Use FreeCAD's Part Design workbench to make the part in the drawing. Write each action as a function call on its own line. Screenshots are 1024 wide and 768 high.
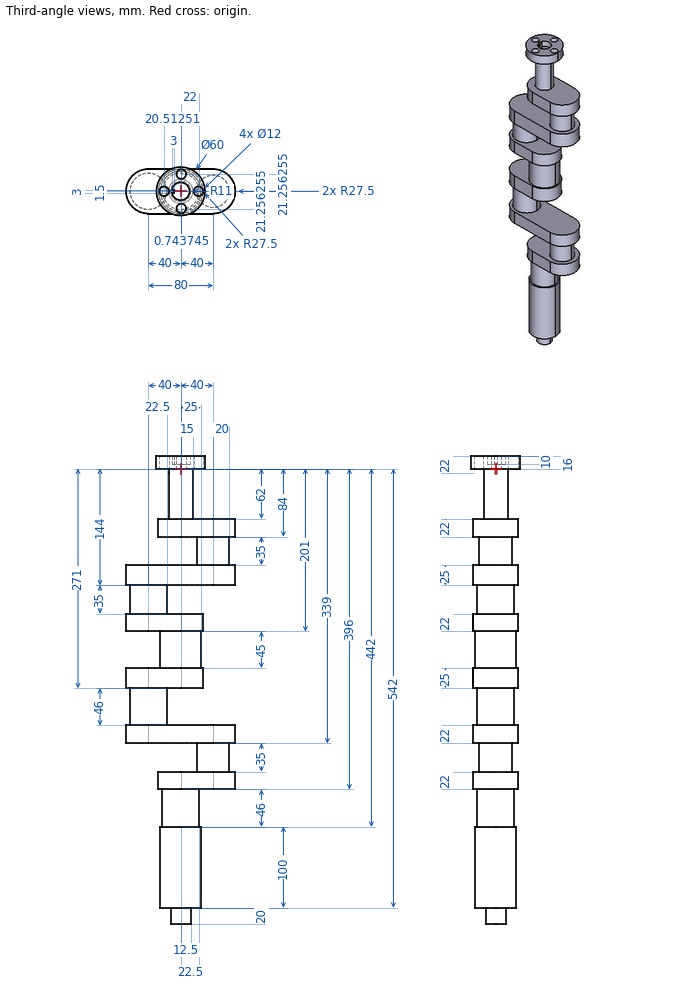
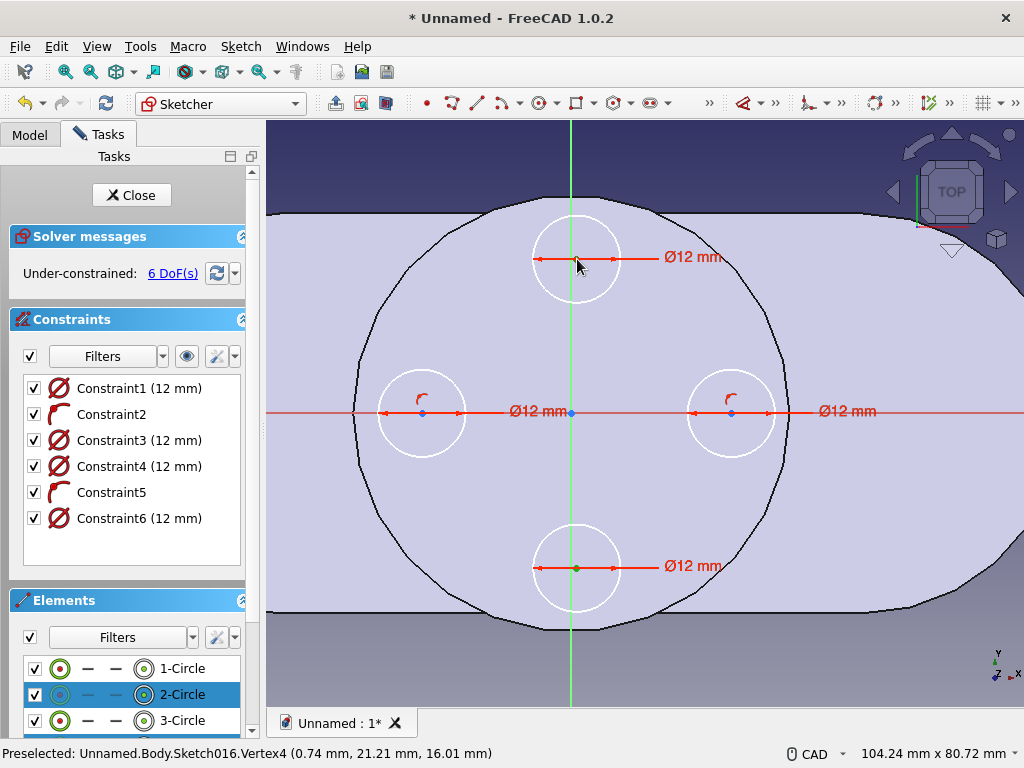
key(v)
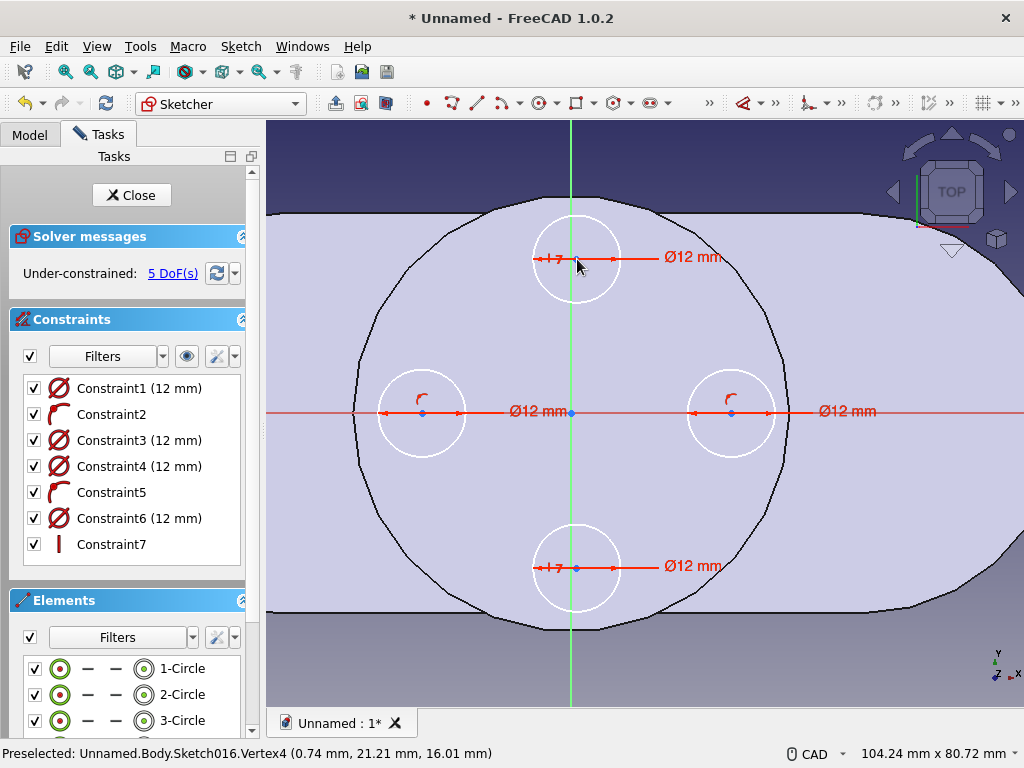
key(d)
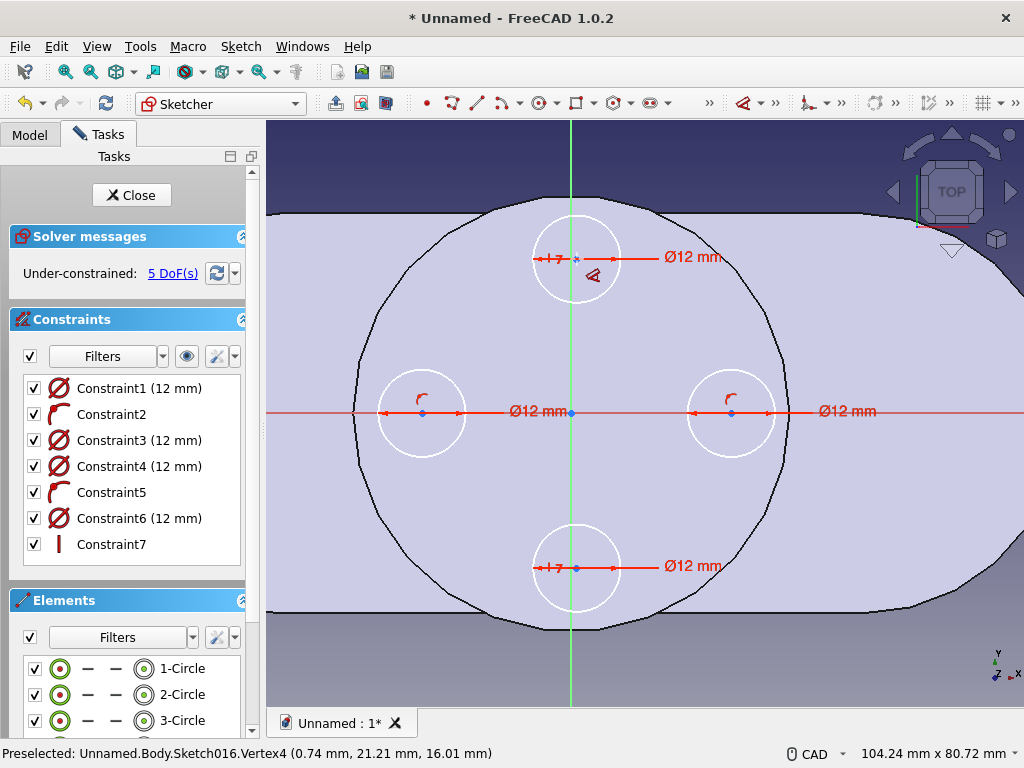
click(731, 413)
click(651, 447)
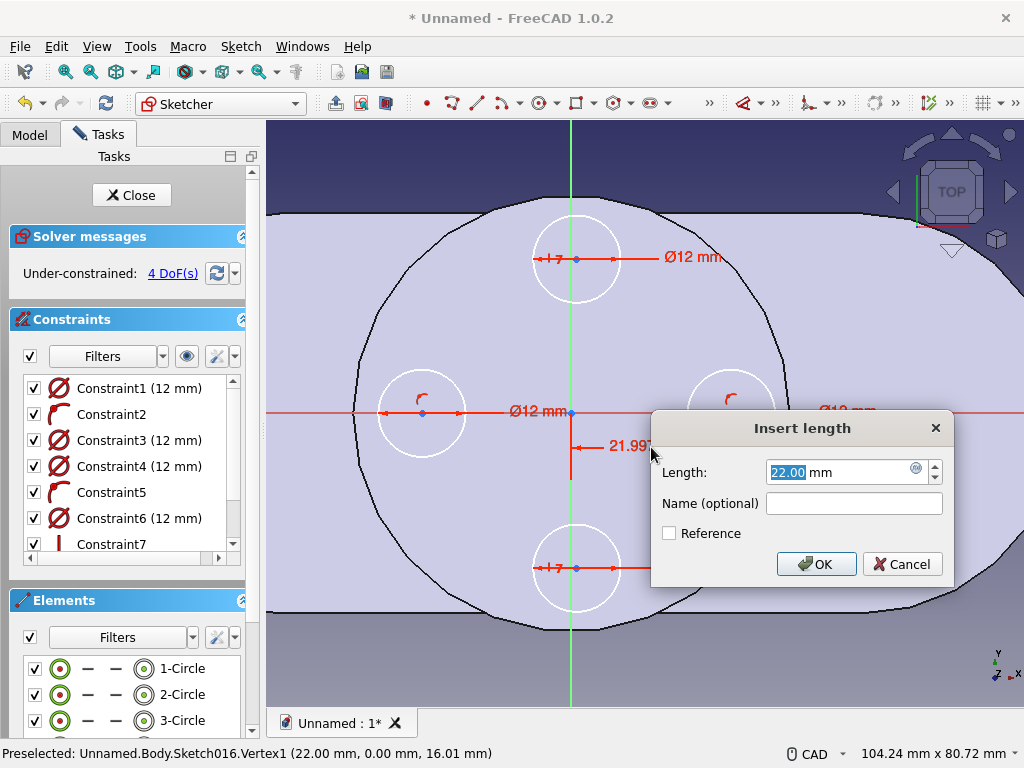
text(22)
key(Return)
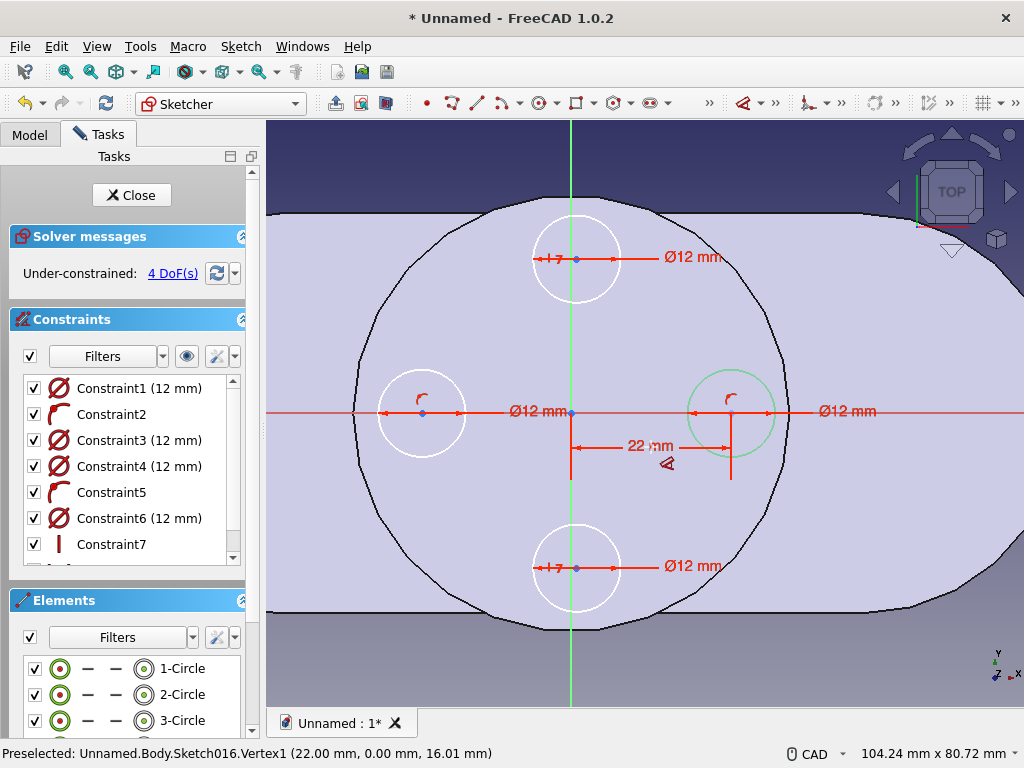
scroll(577, 568, up, 10)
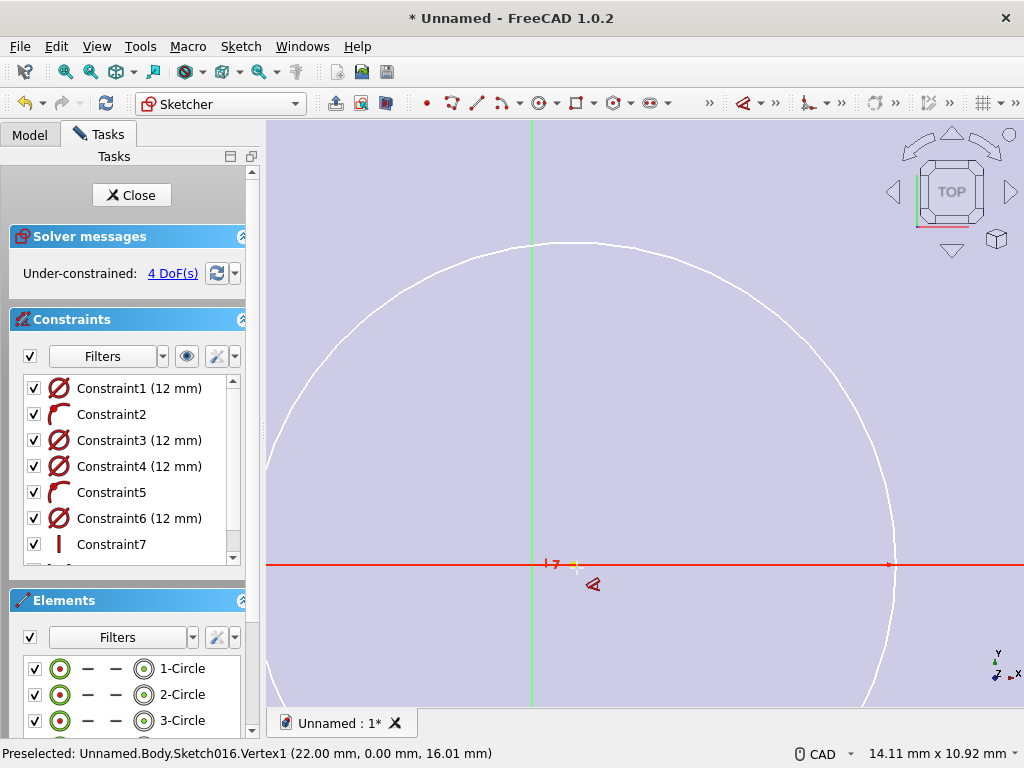
click(573, 565)
click(553, 599)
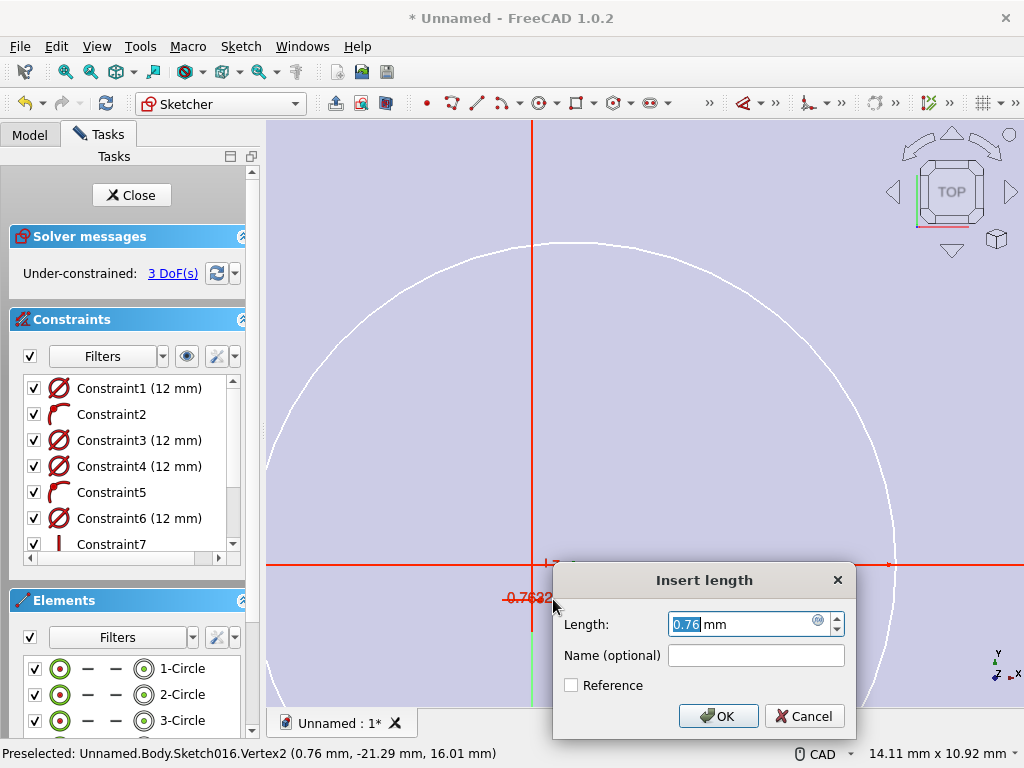
text(0.743745)
key(Return)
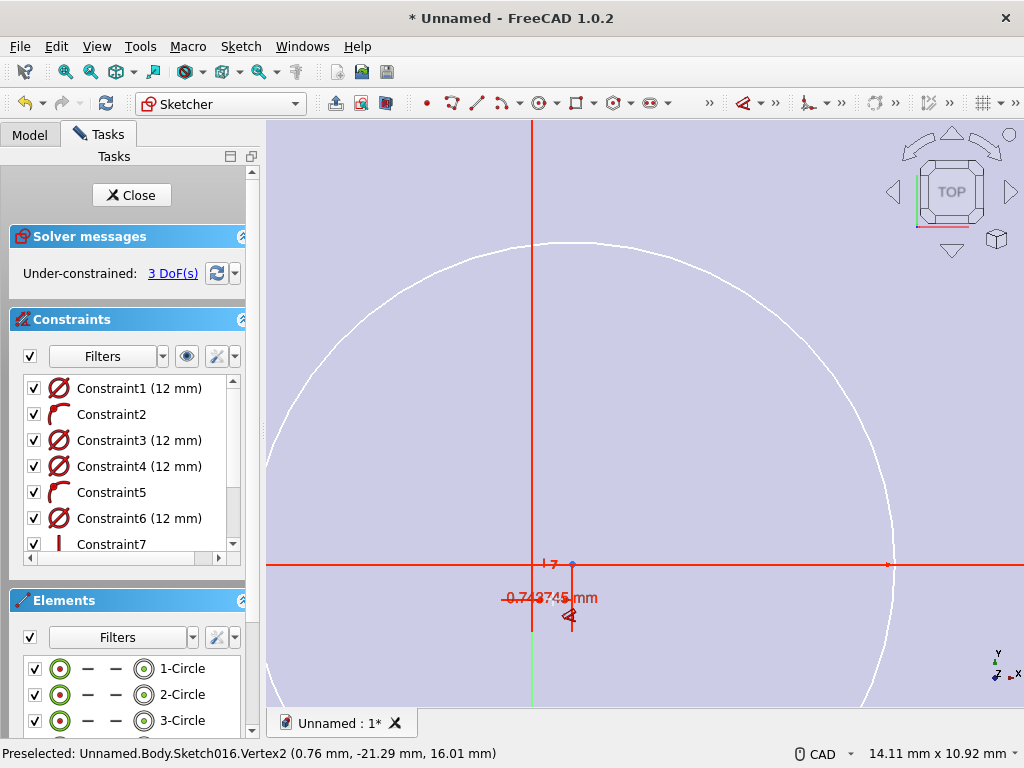
scroll(577, 569, down, 10)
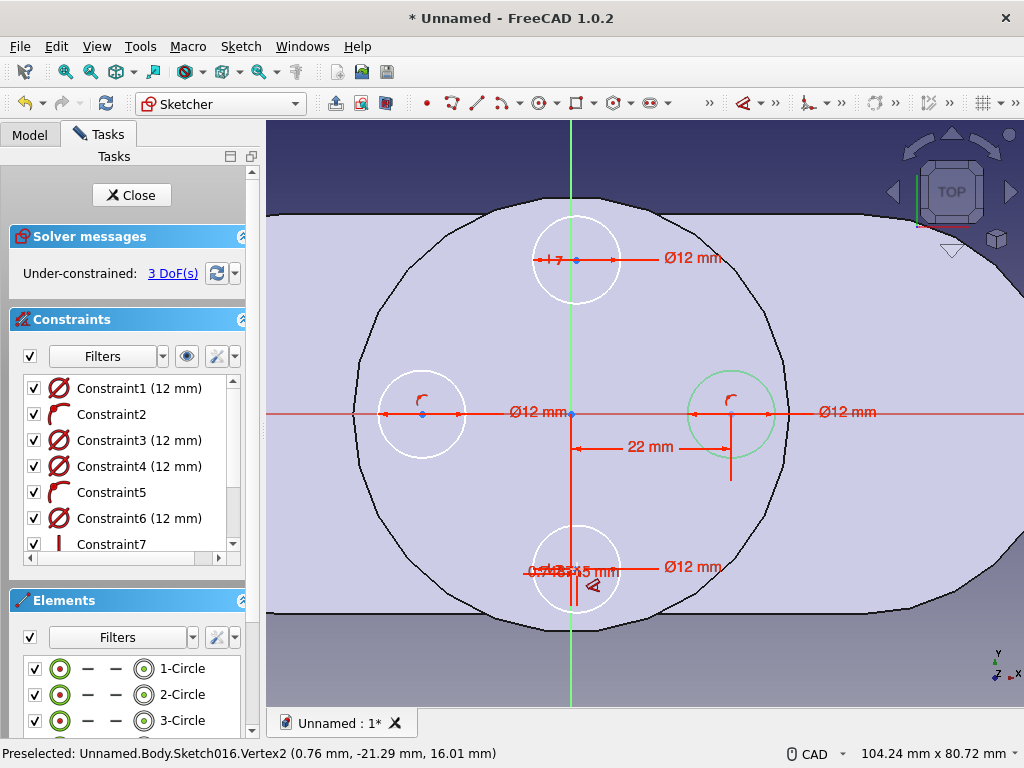
click(422, 414)
click(497, 448)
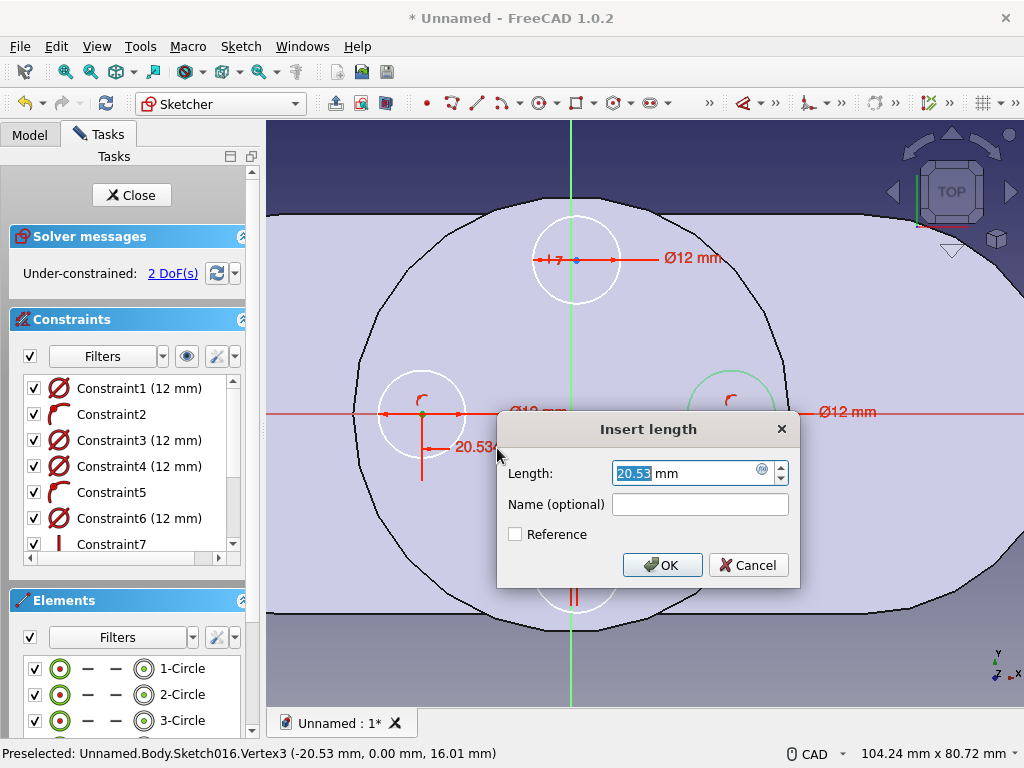
text(20.51251)
key(Return)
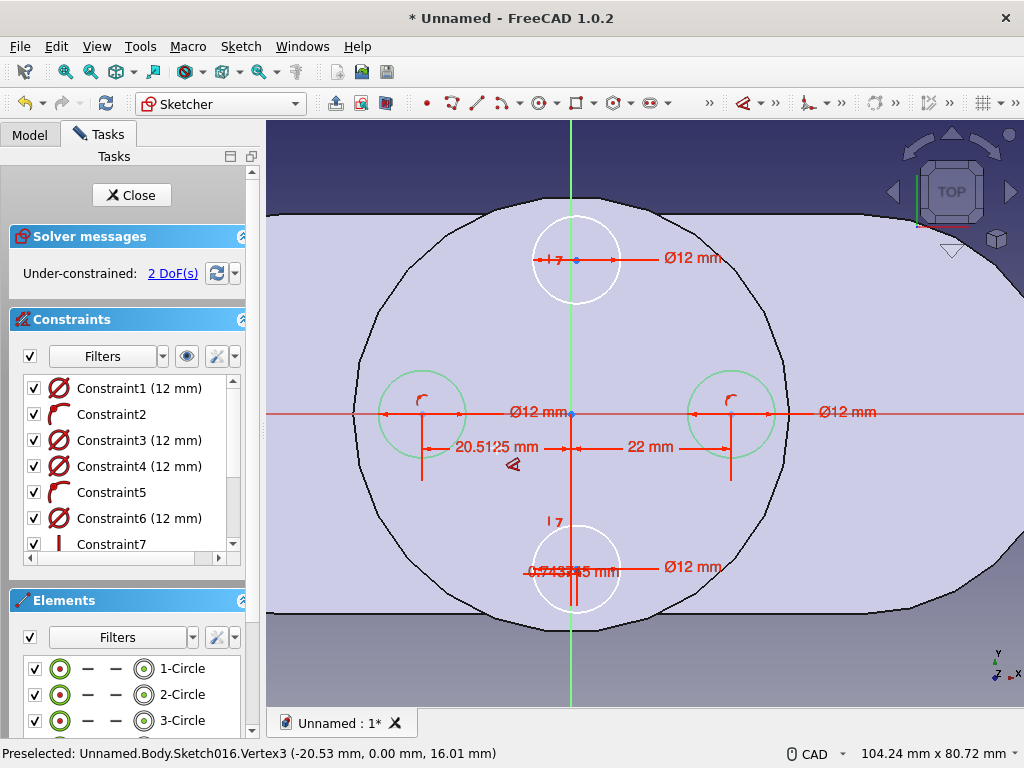
click(577, 569)
click(537, 492)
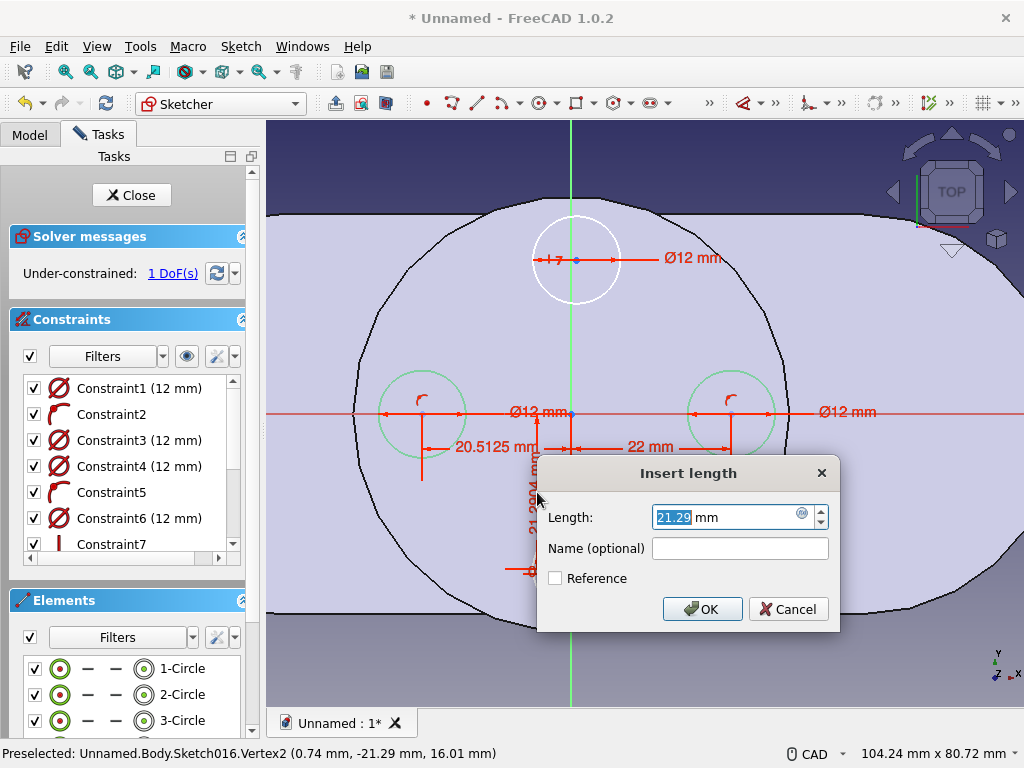
text(21.256255)
key(Return)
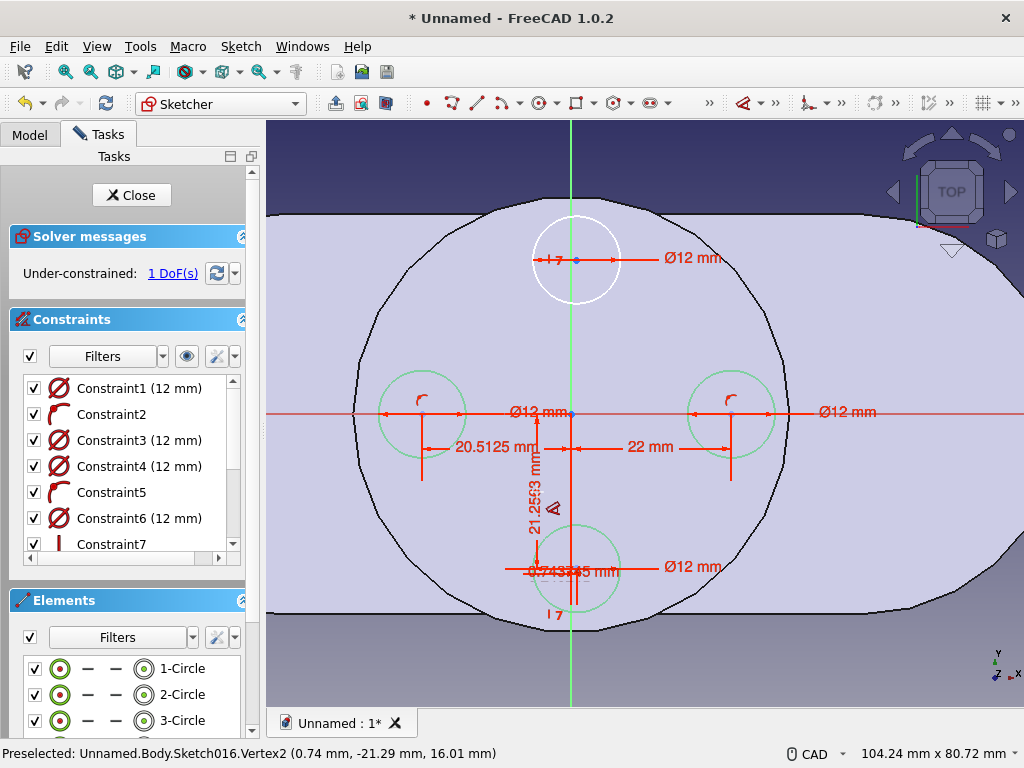
click(577, 260)
click(537, 337)